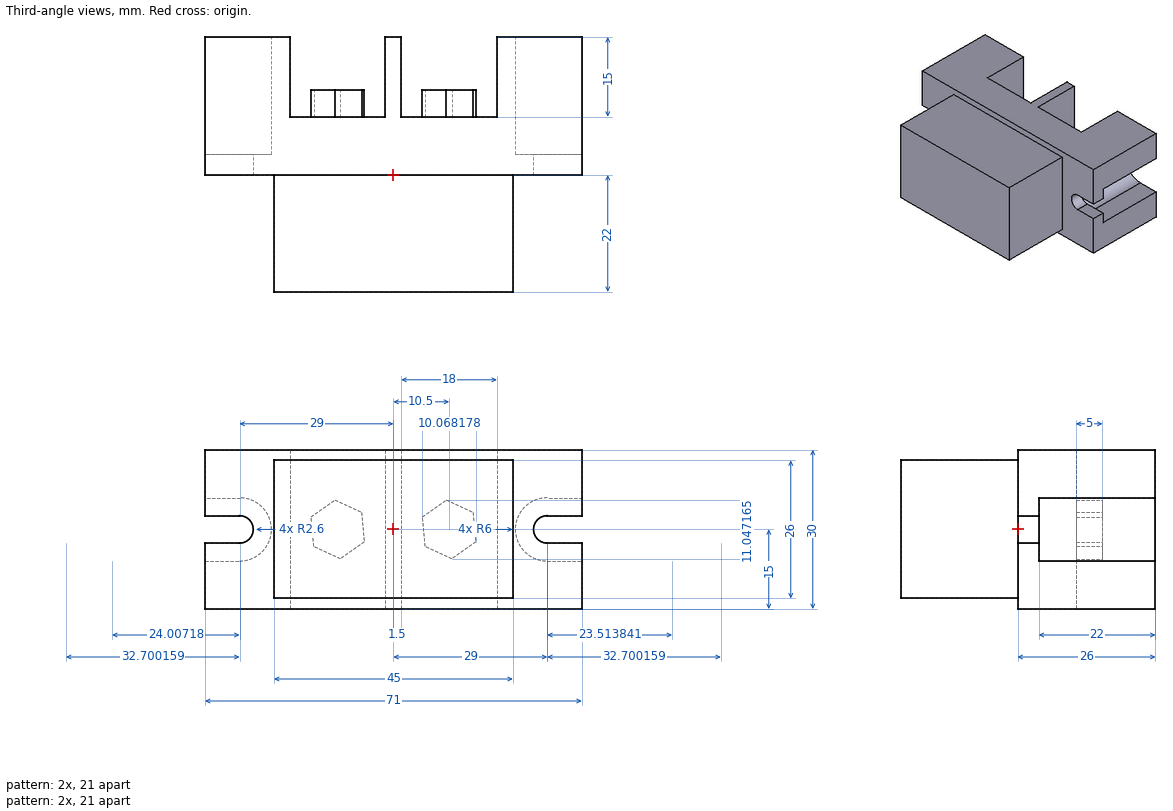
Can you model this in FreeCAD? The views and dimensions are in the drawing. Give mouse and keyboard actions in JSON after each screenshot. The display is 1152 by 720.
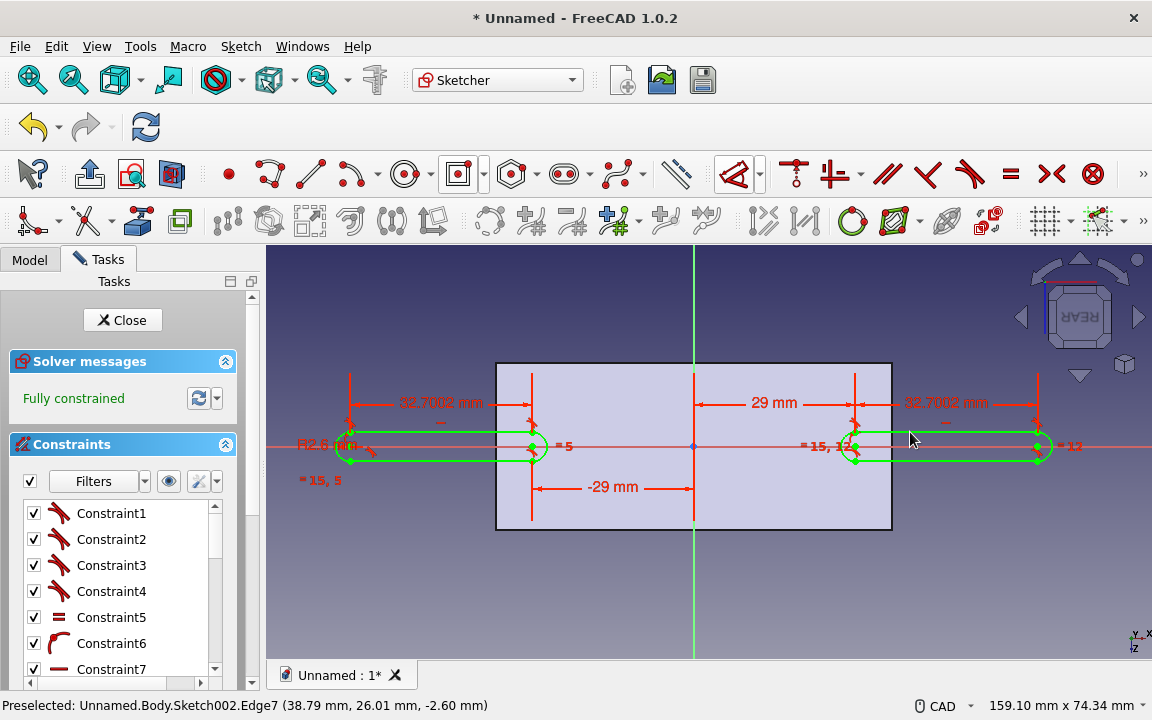
{"action": "left_click", "coordinate": [123, 320]}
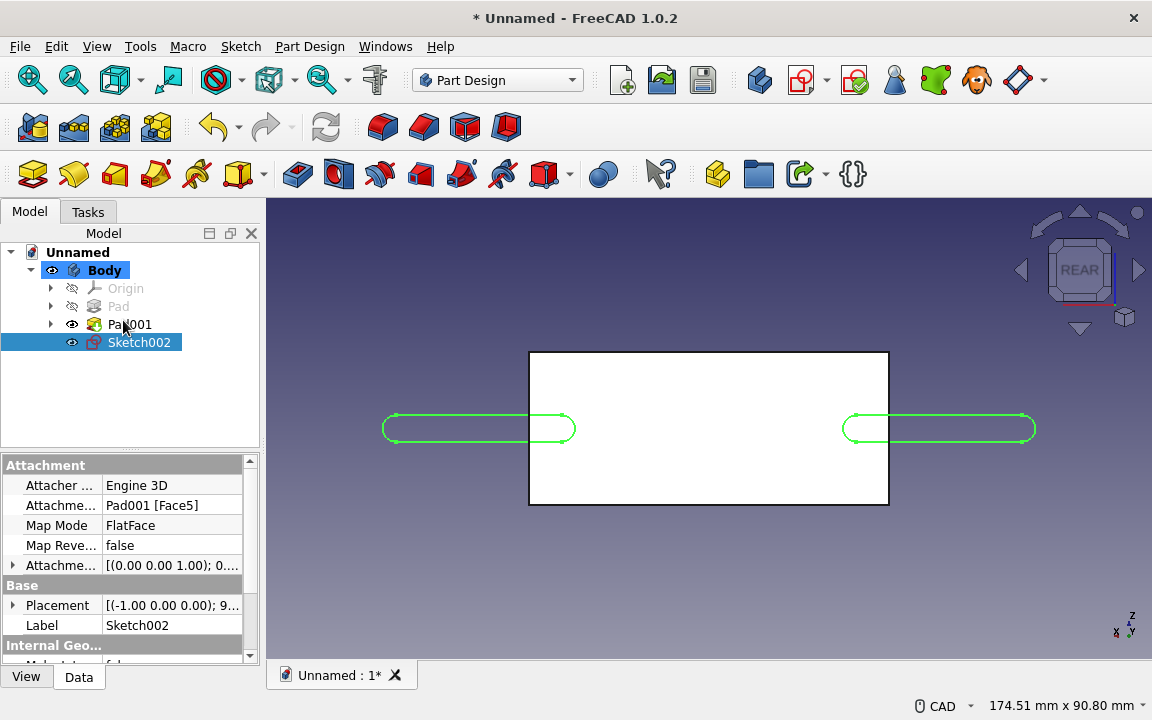
{"action": "left_click", "coordinate": [298, 174]}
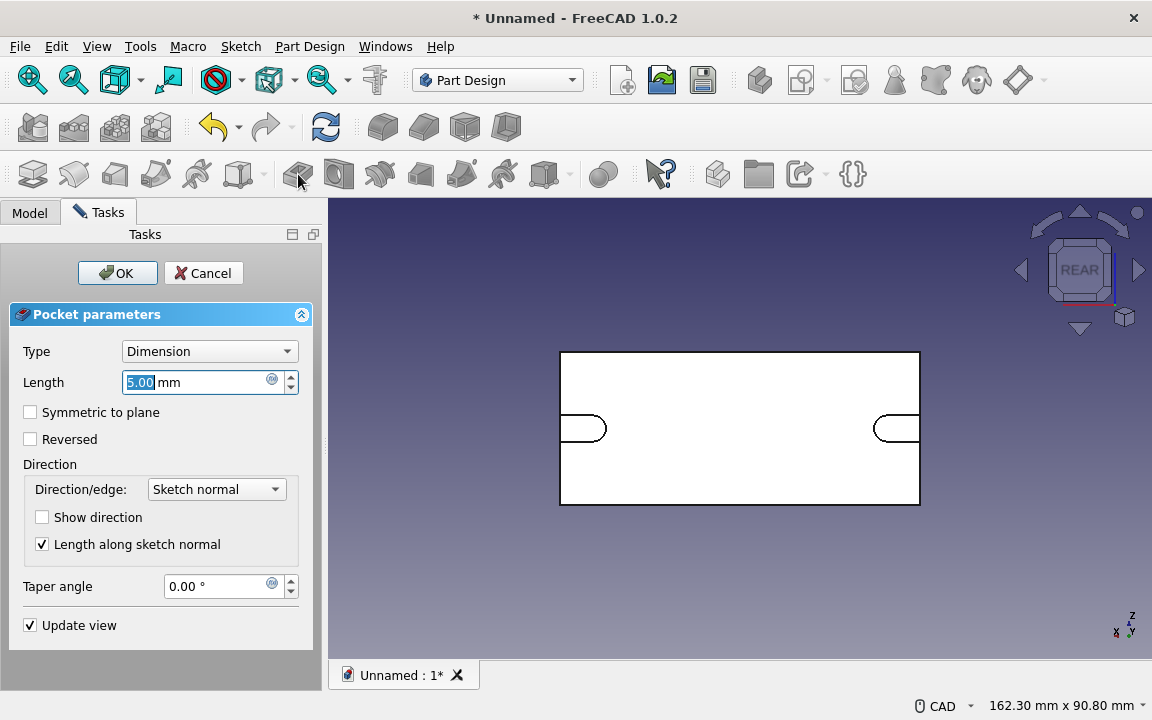
{"action": "left_click", "coordinate": [210, 352]}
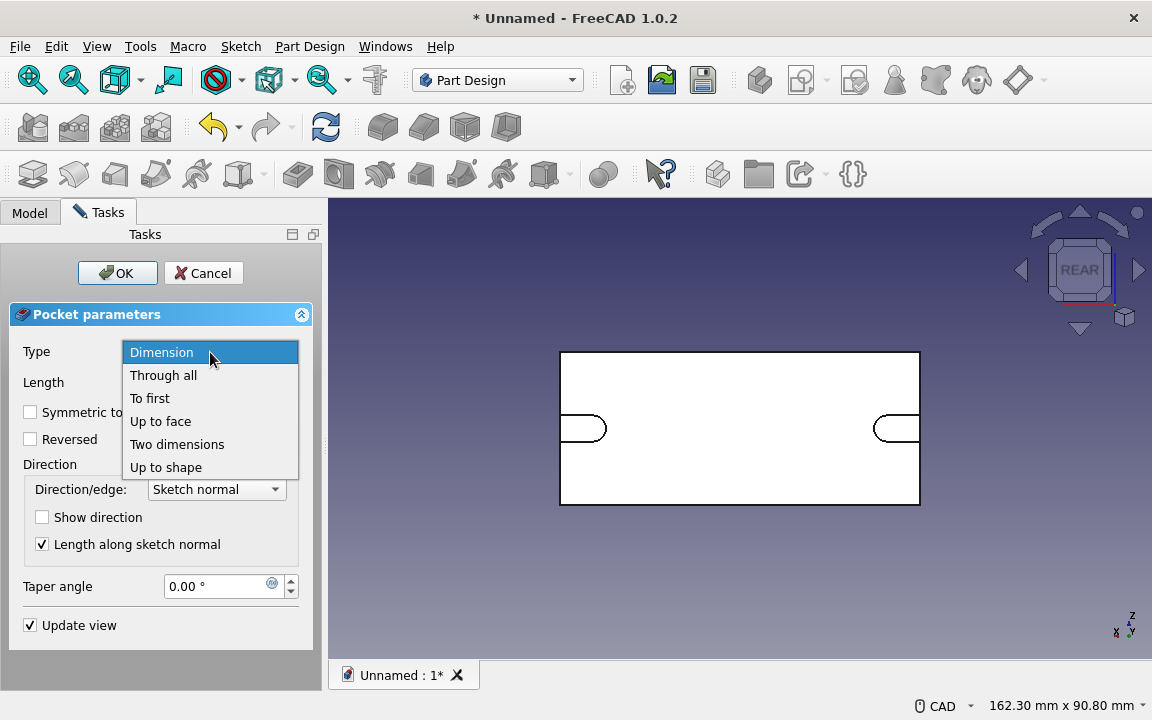
{"action": "left_click", "coordinate": [208, 376]}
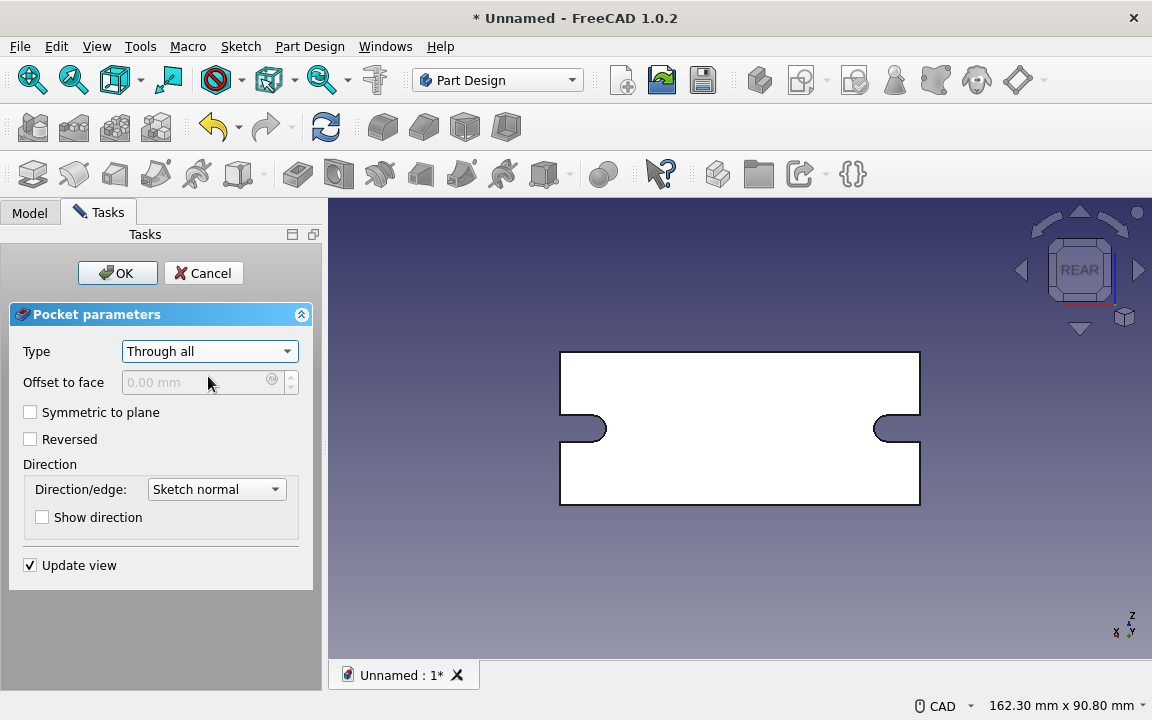
{"action": "left_click", "coordinate": [118, 273]}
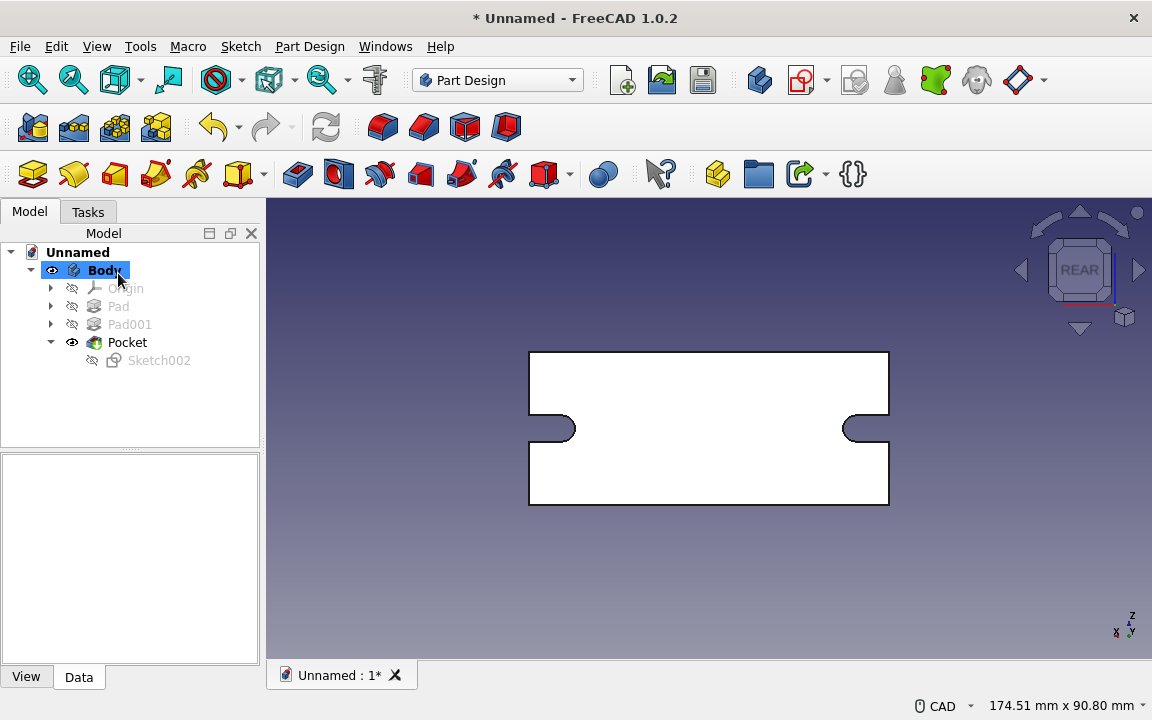
{"action": "left_click", "coordinate": [33, 80]}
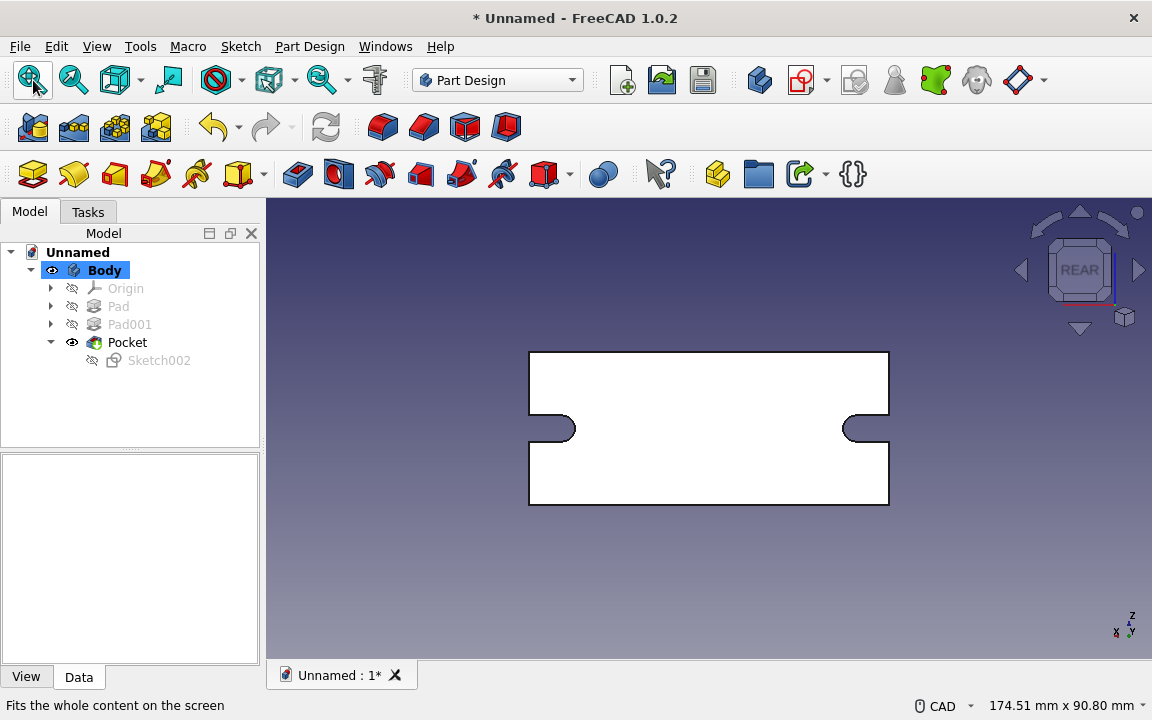
{"action": "left_click", "coordinate": [658, 427]}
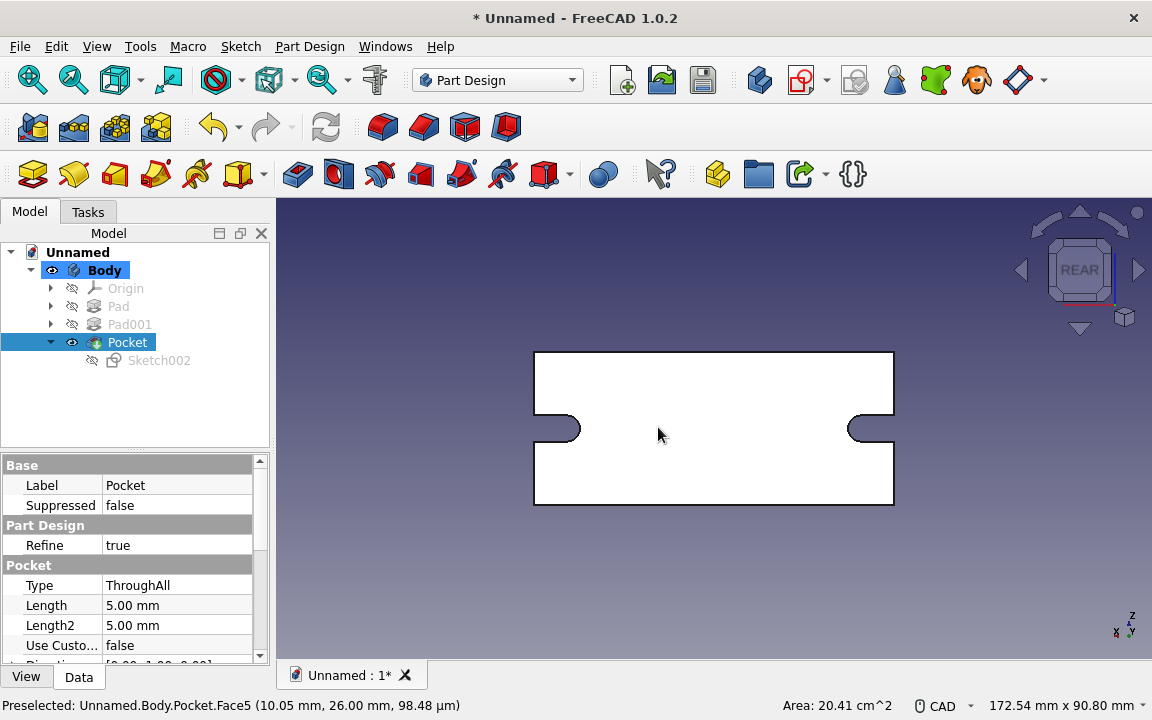
{"action": "left_click", "coordinate": [800, 80]}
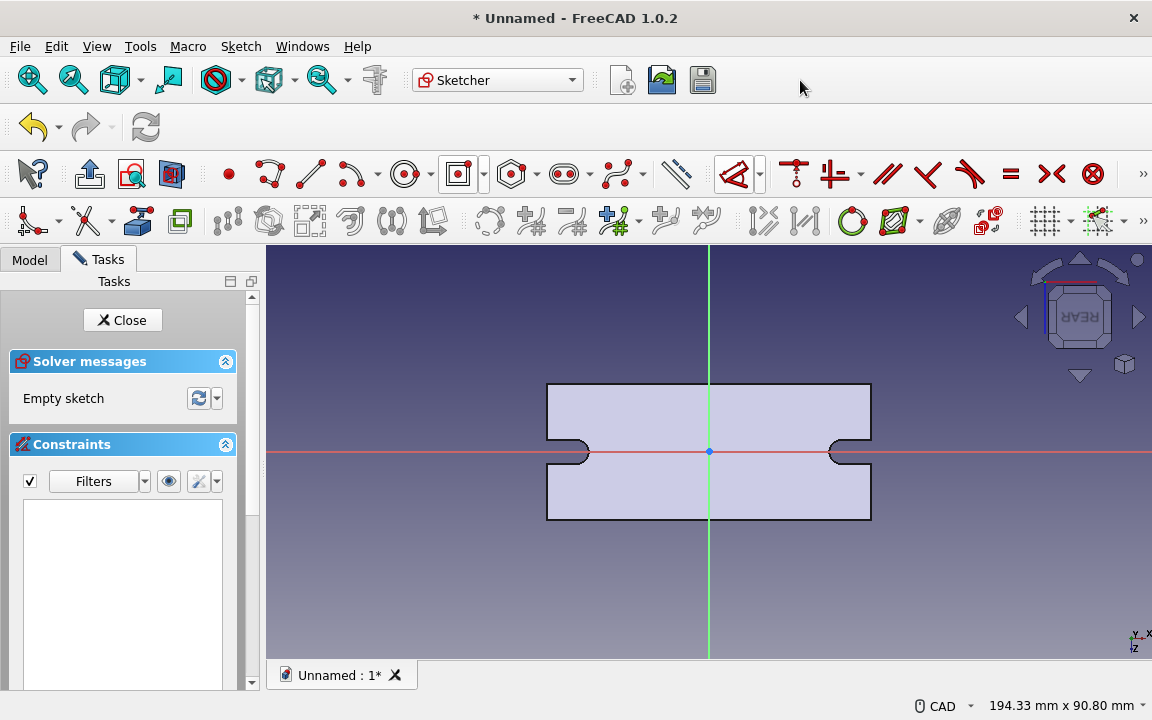
{"action": "scroll", "coordinate": [336, 452], "scroll_direction": "down", "scroll_amount": 1}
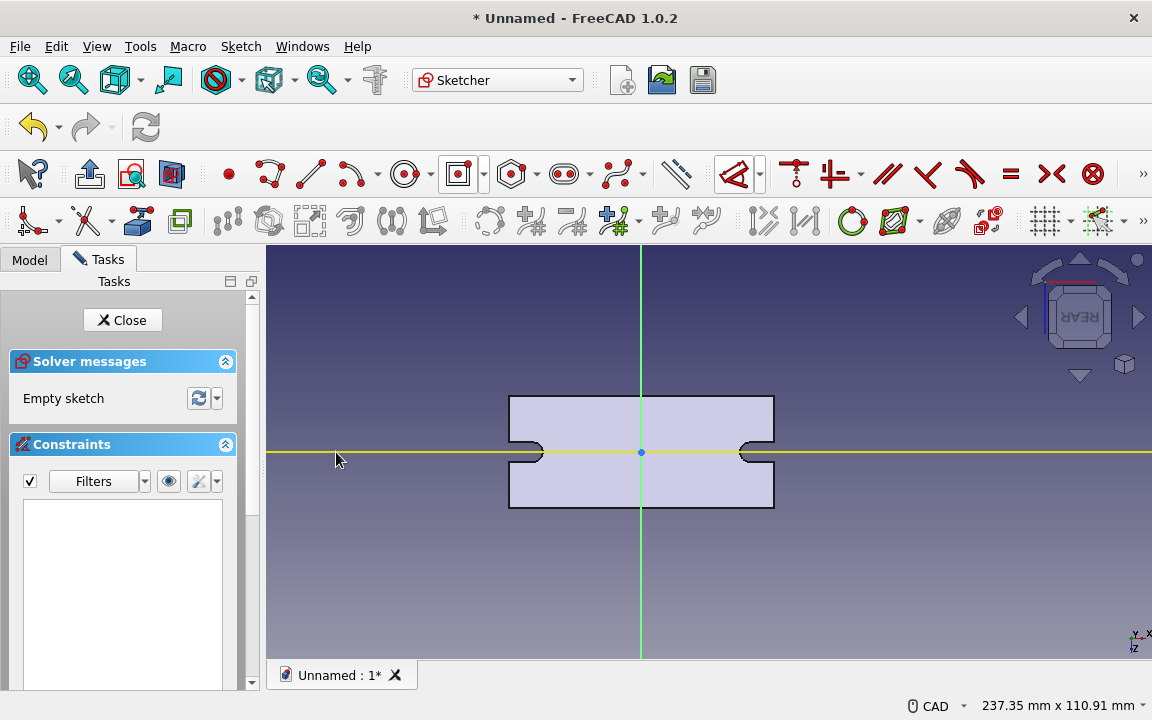
{"action": "key", "text": "g s"}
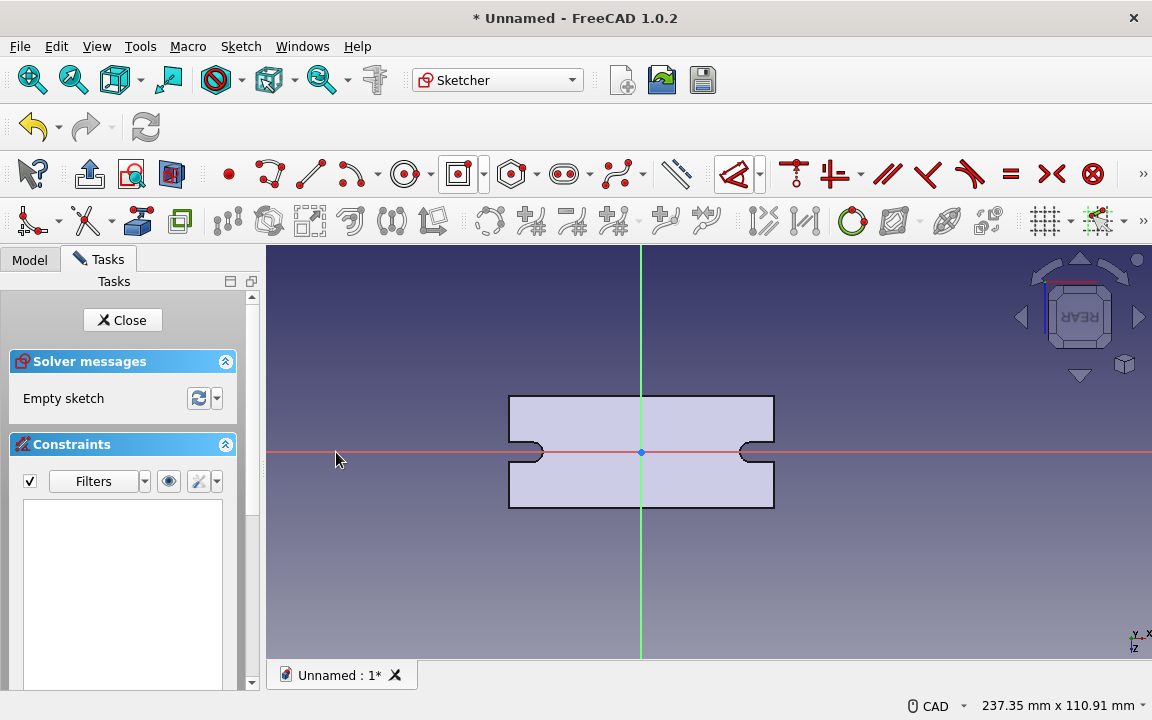
{"action": "left_click", "coordinate": [750, 452]}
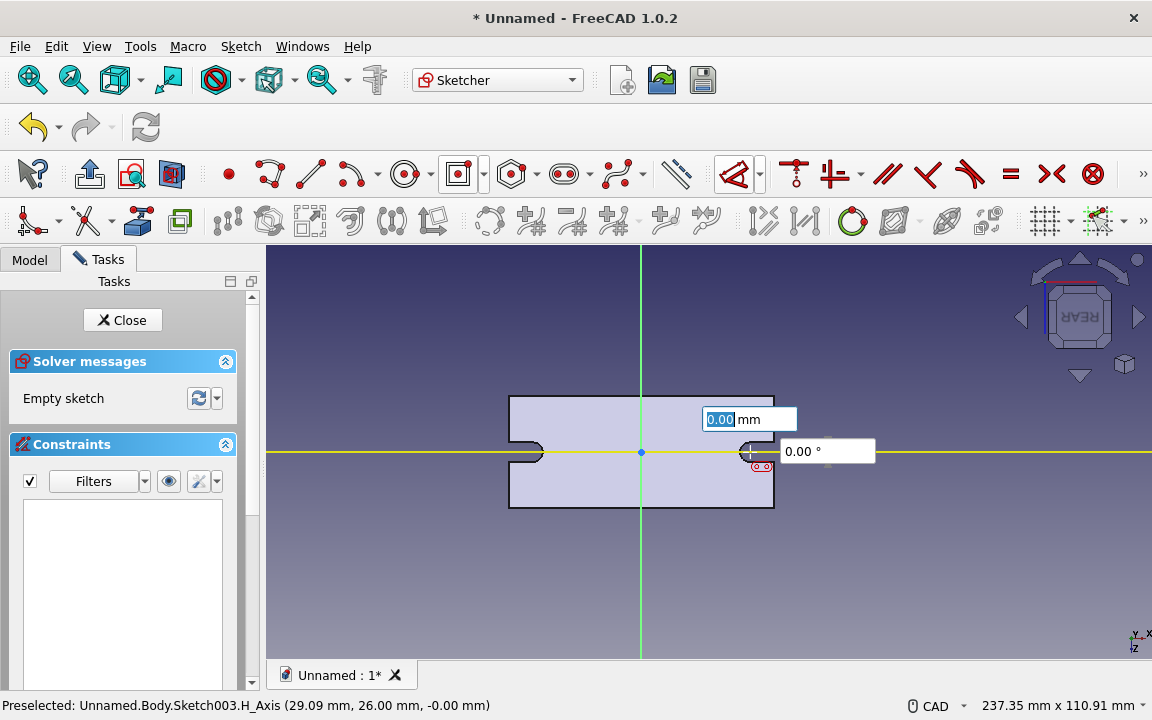
{"action": "left_click", "coordinate": [837, 443]}